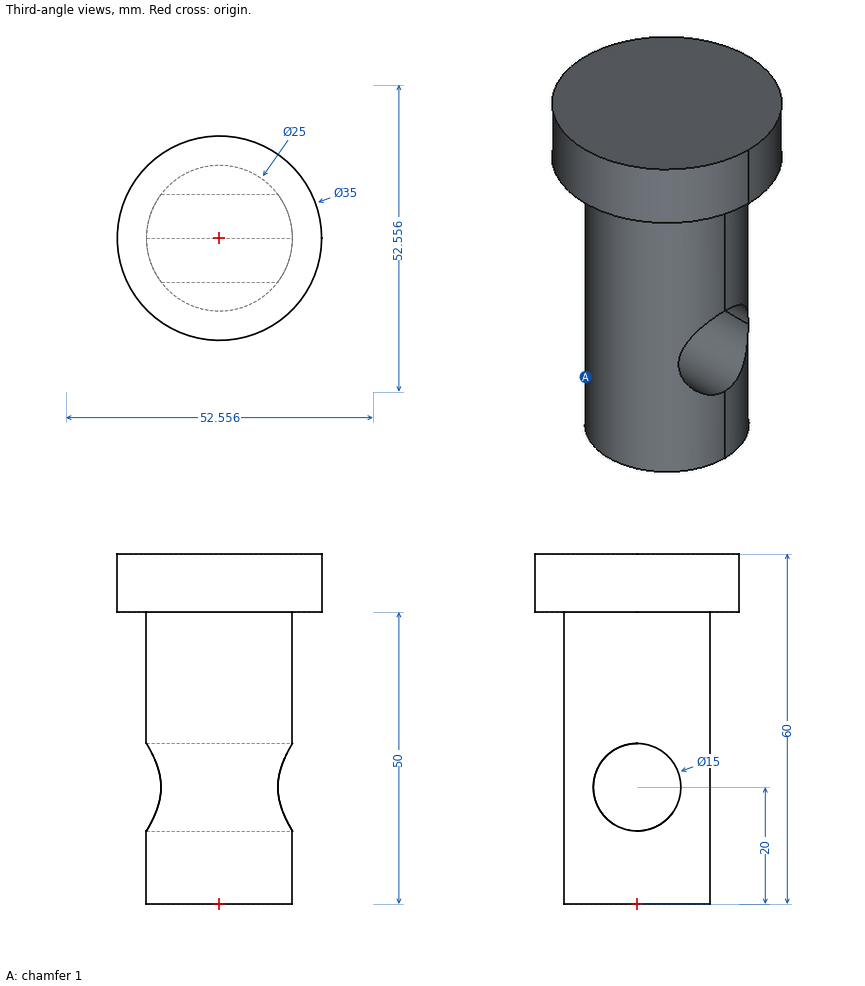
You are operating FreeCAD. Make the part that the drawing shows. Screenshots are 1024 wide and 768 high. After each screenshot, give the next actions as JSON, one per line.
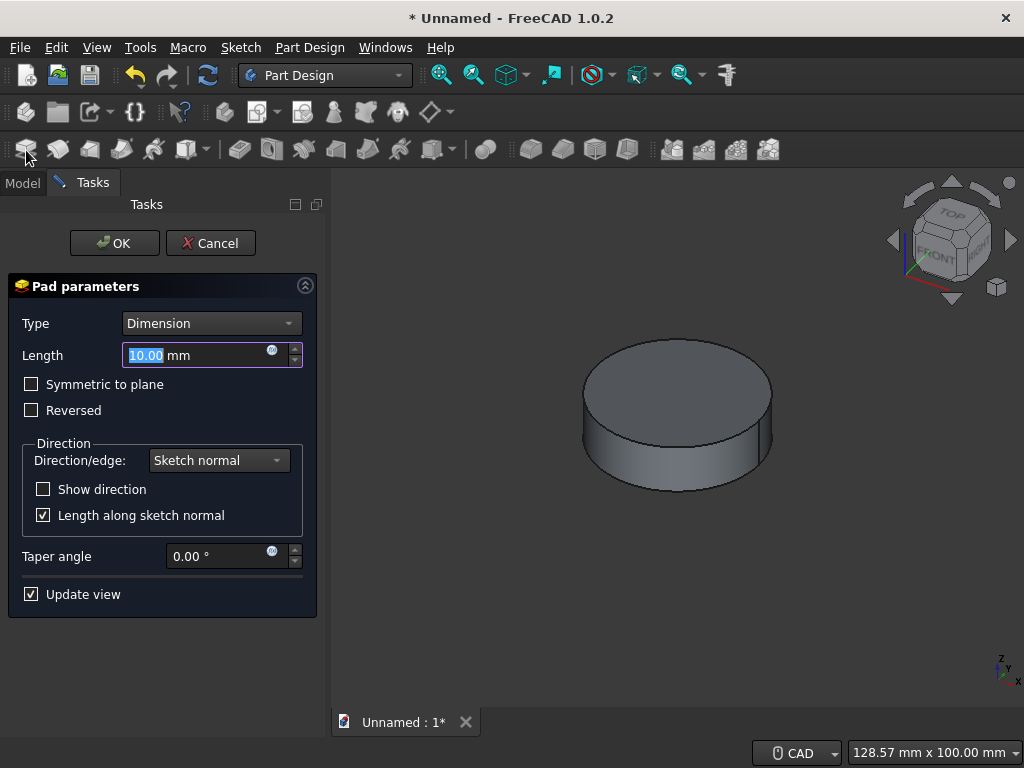
{"action": "type", "text": "60"}
{"action": "key", "text": "Tab"}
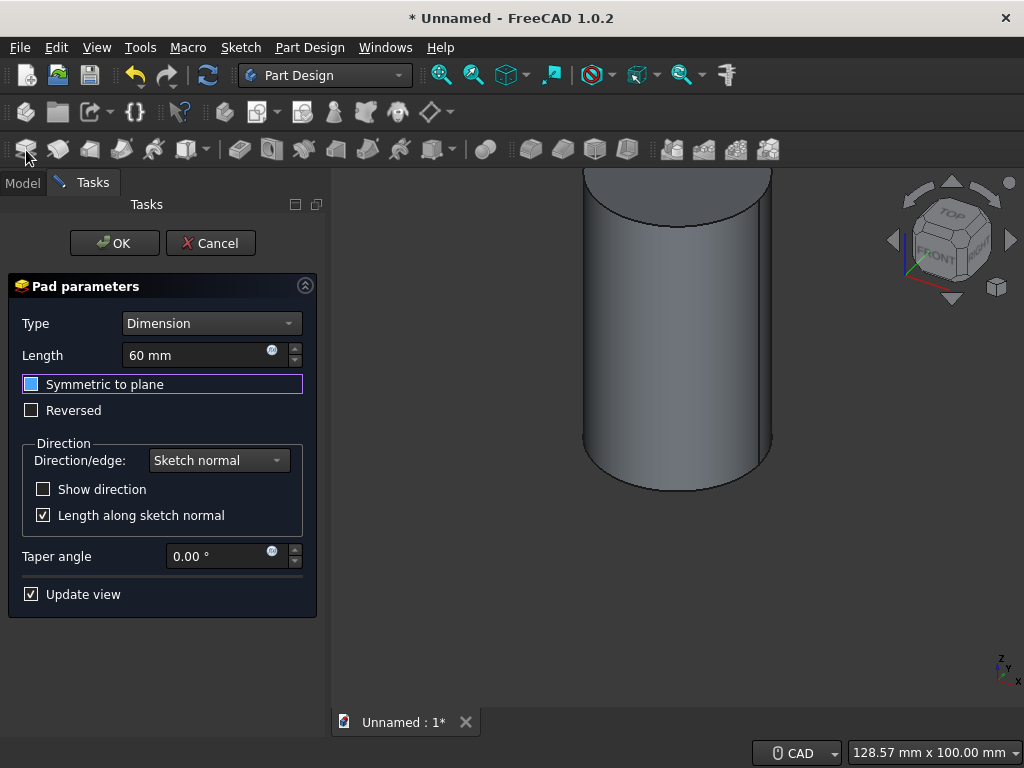
{"action": "left_click", "coordinate": [115, 243]}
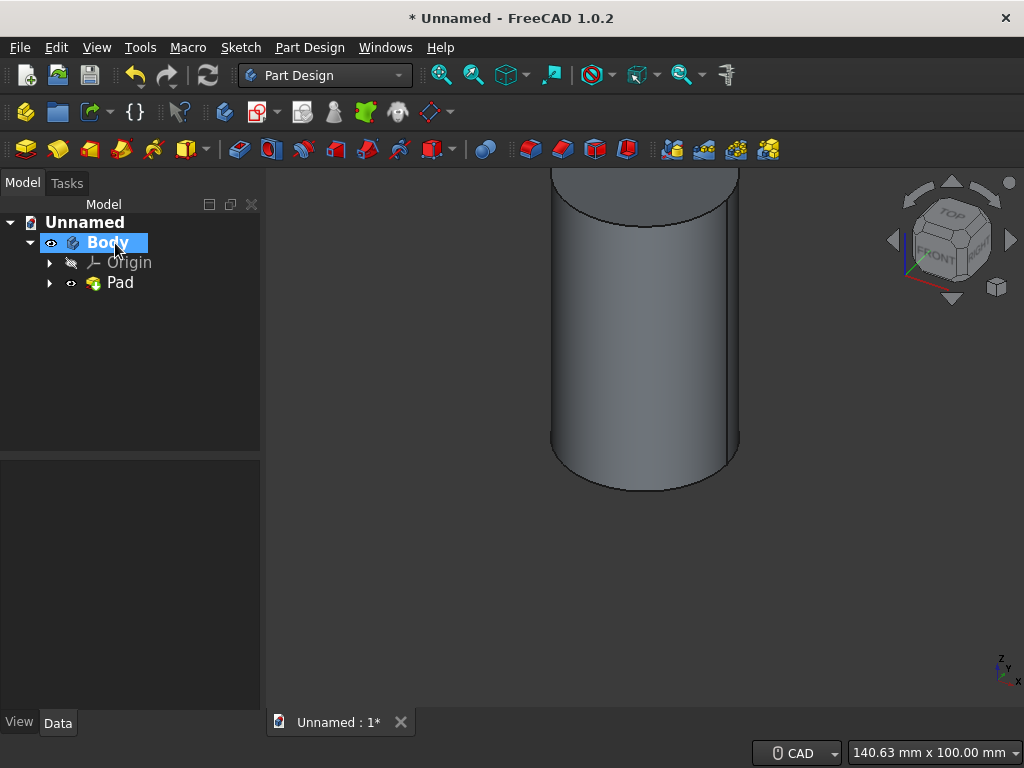
{"action": "left_click", "coordinate": [442, 76]}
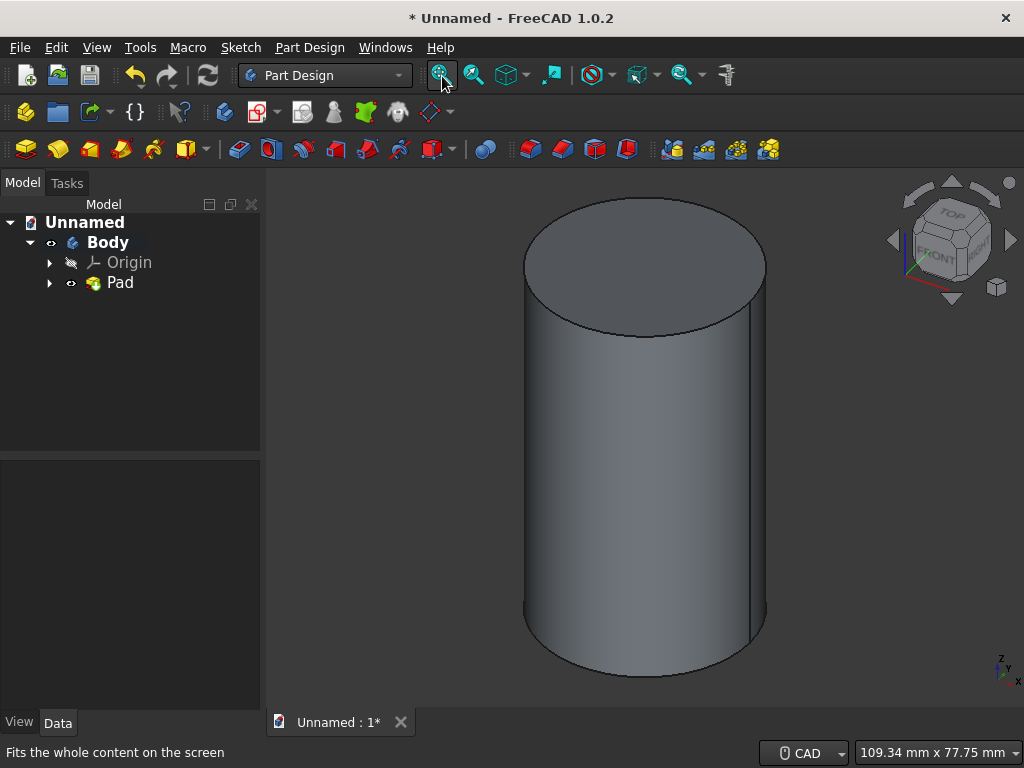
{"action": "key", "text": "0"}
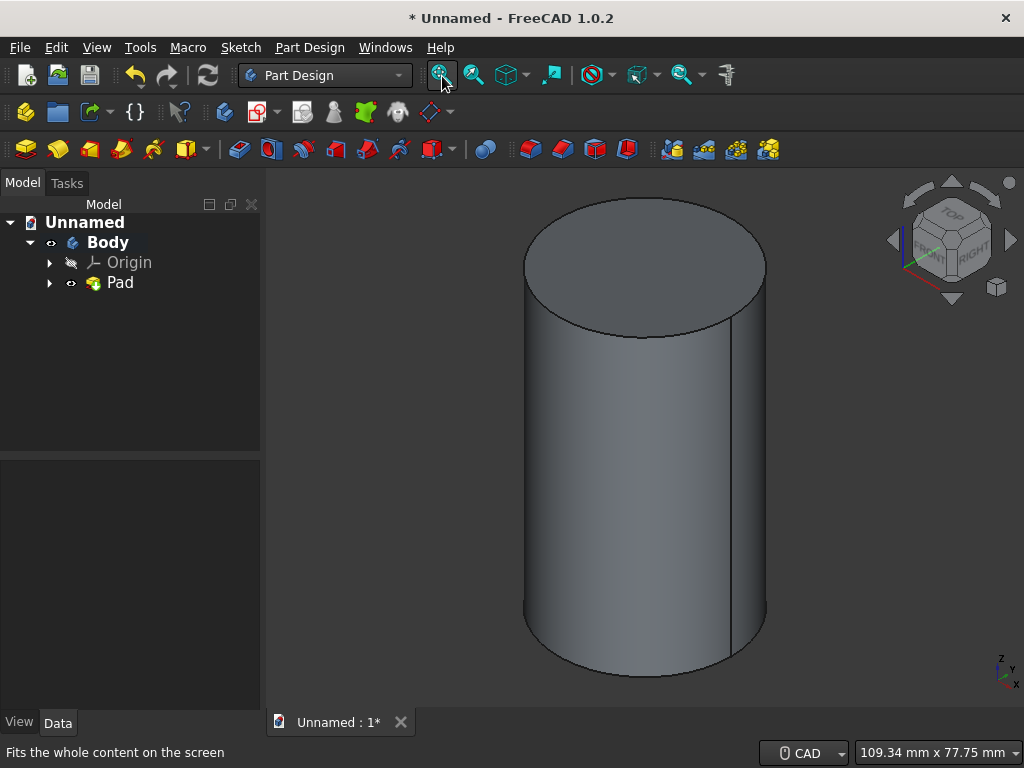
{"action": "left_click", "coordinate": [745, 646]}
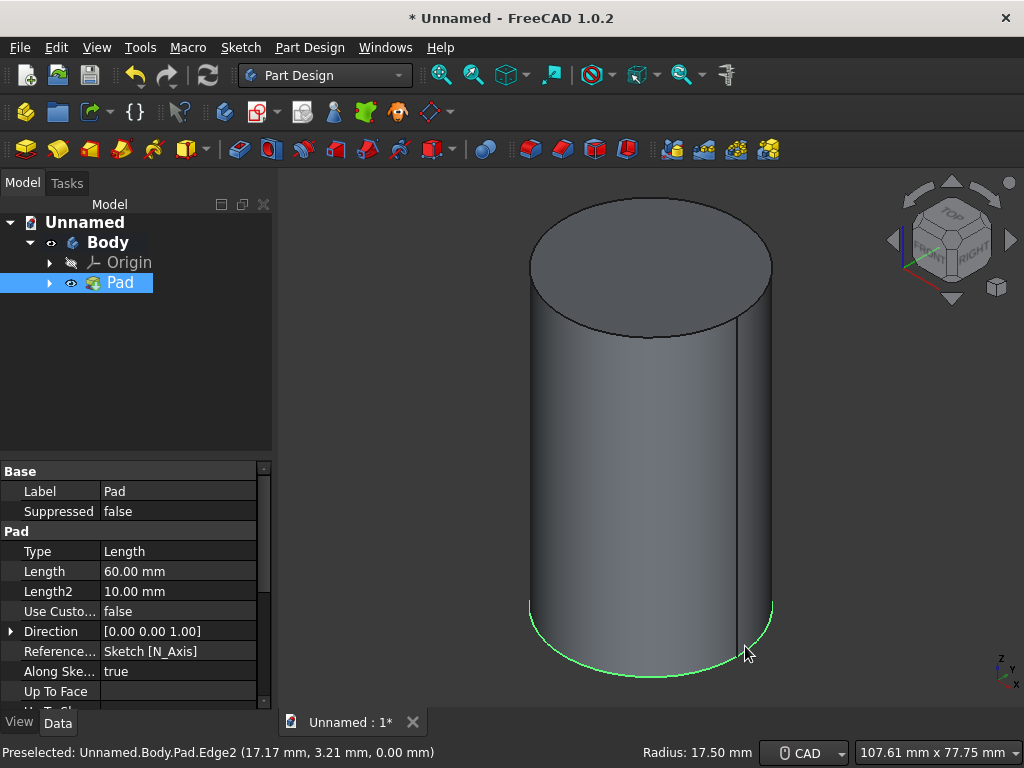
{"action": "left_click", "coordinate": [564, 150]}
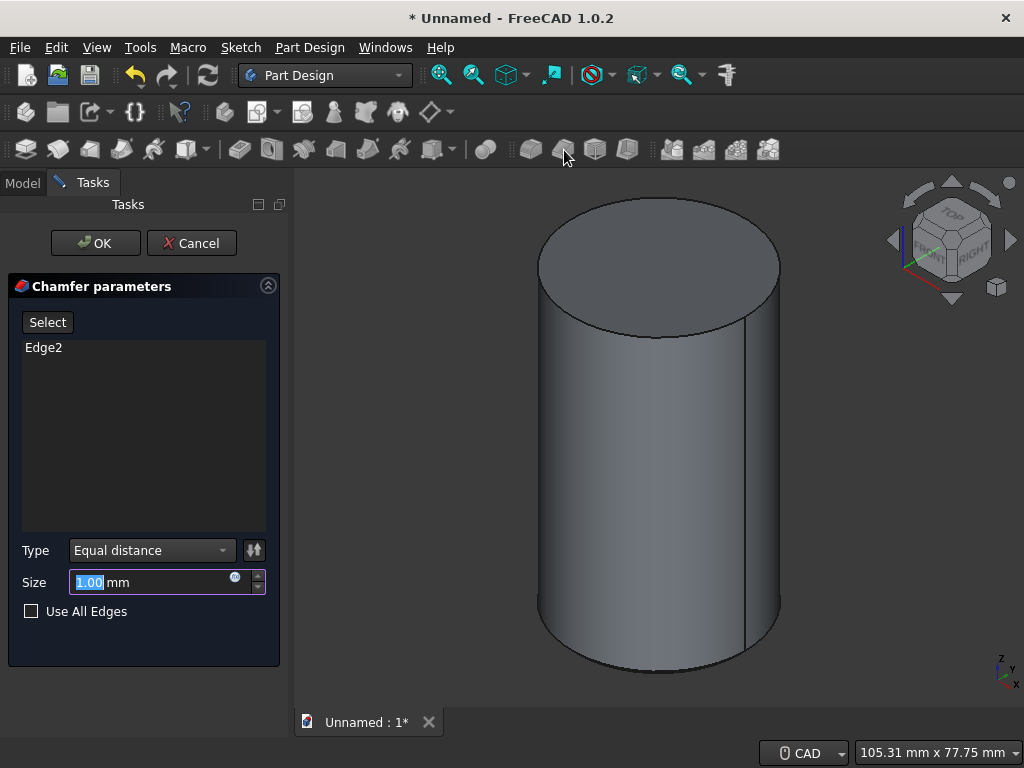
{"action": "type", "text": "1"}
{"action": "key", "text": "Tab"}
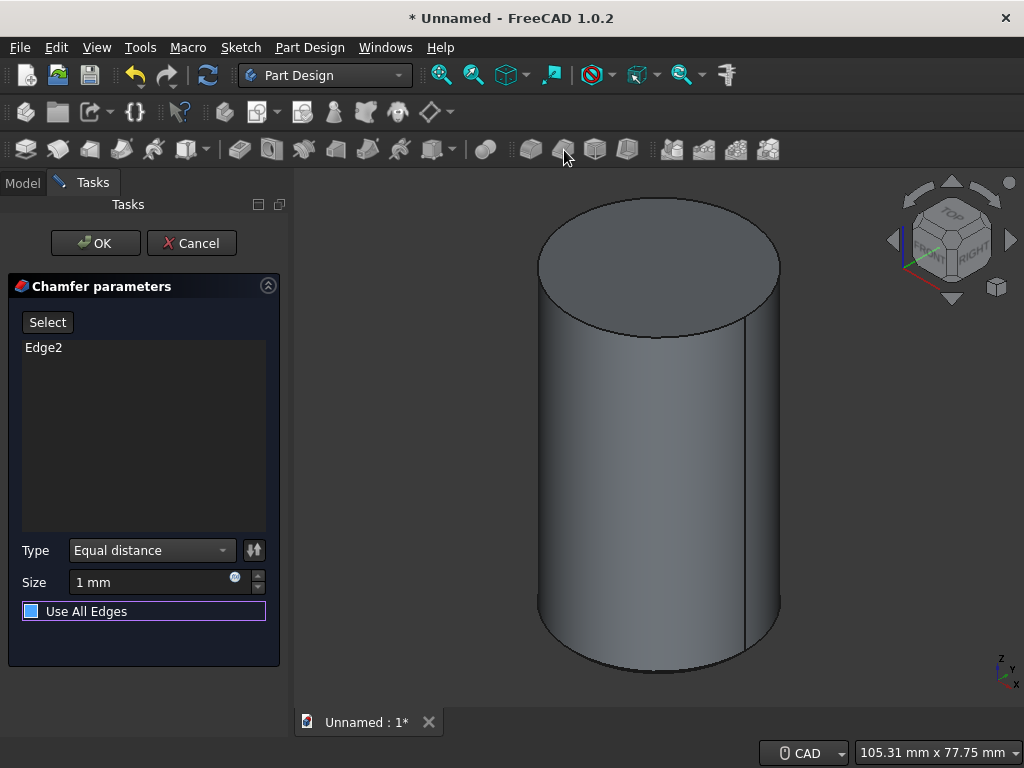
{"action": "left_click", "coordinate": [96, 243]}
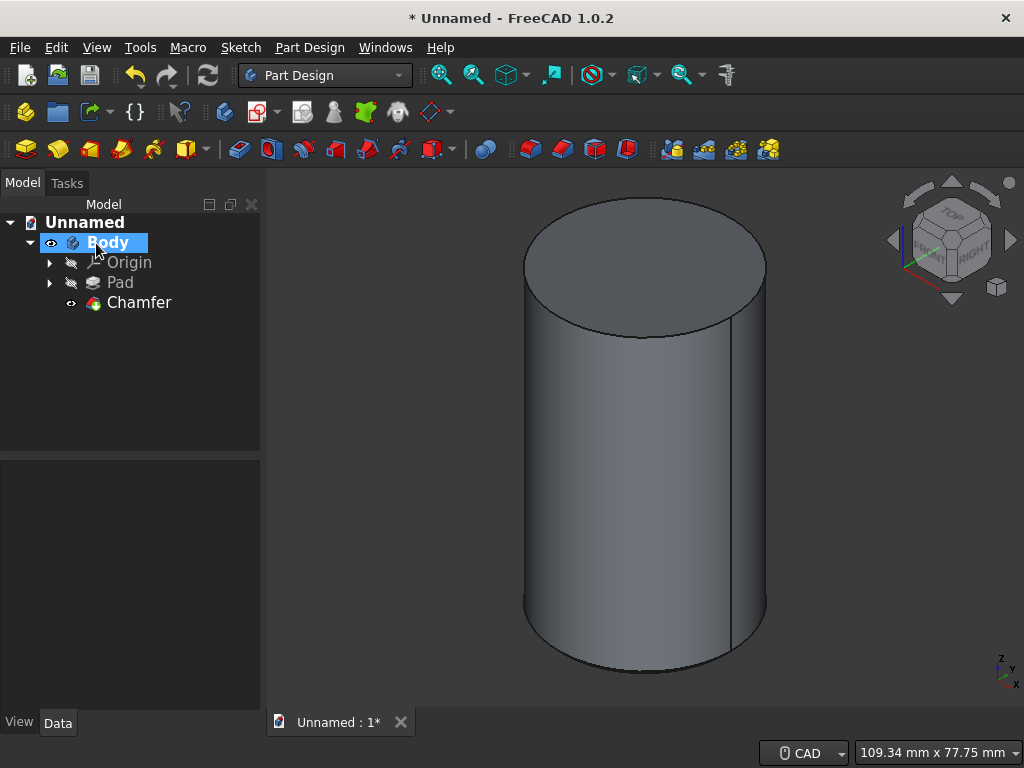
{"action": "left_click", "coordinate": [258, 112]}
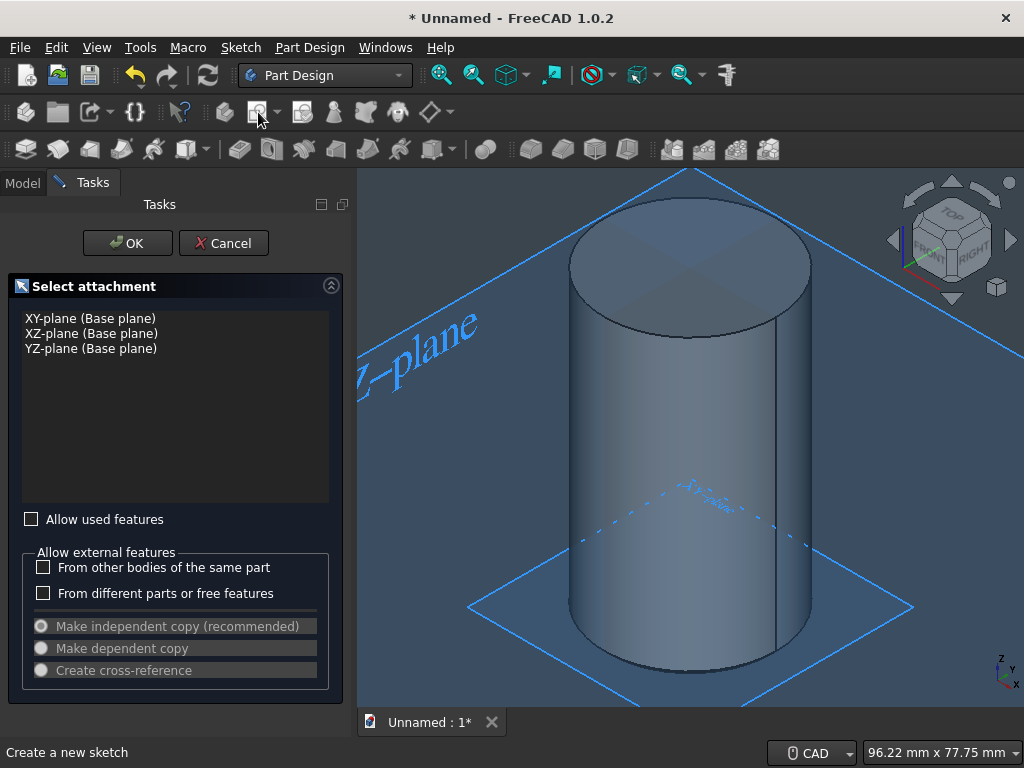
{"action": "left_click", "coordinate": [82, 348]}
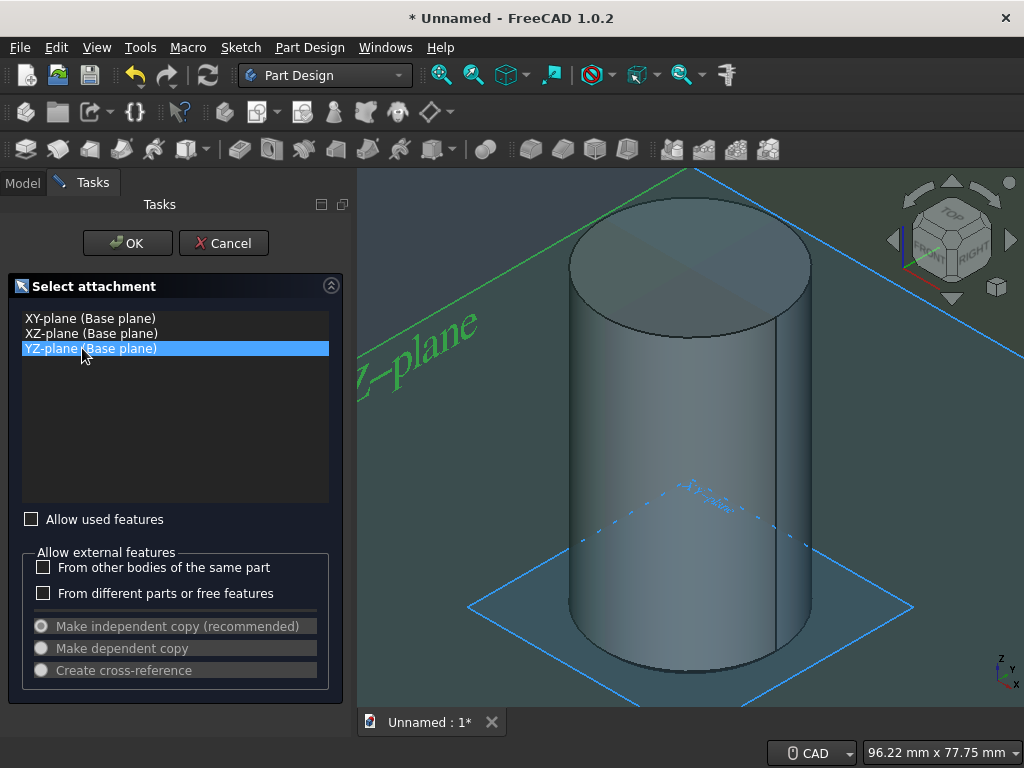
{"action": "left_click", "coordinate": [128, 243]}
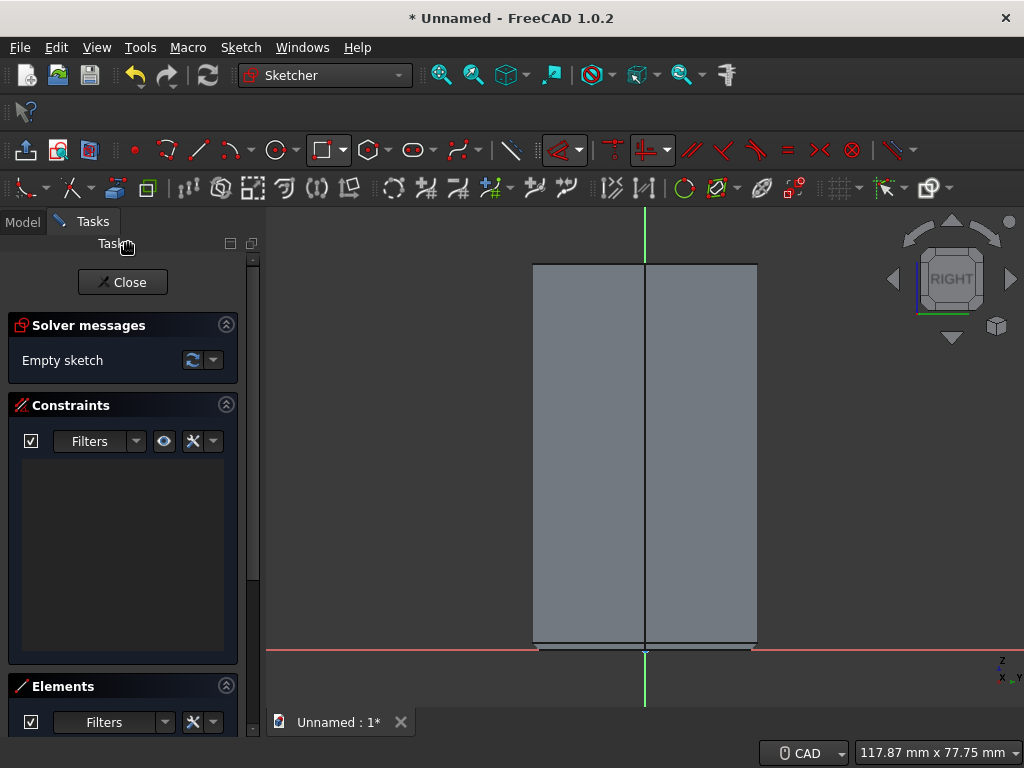
{"action": "key", "text": "q s"}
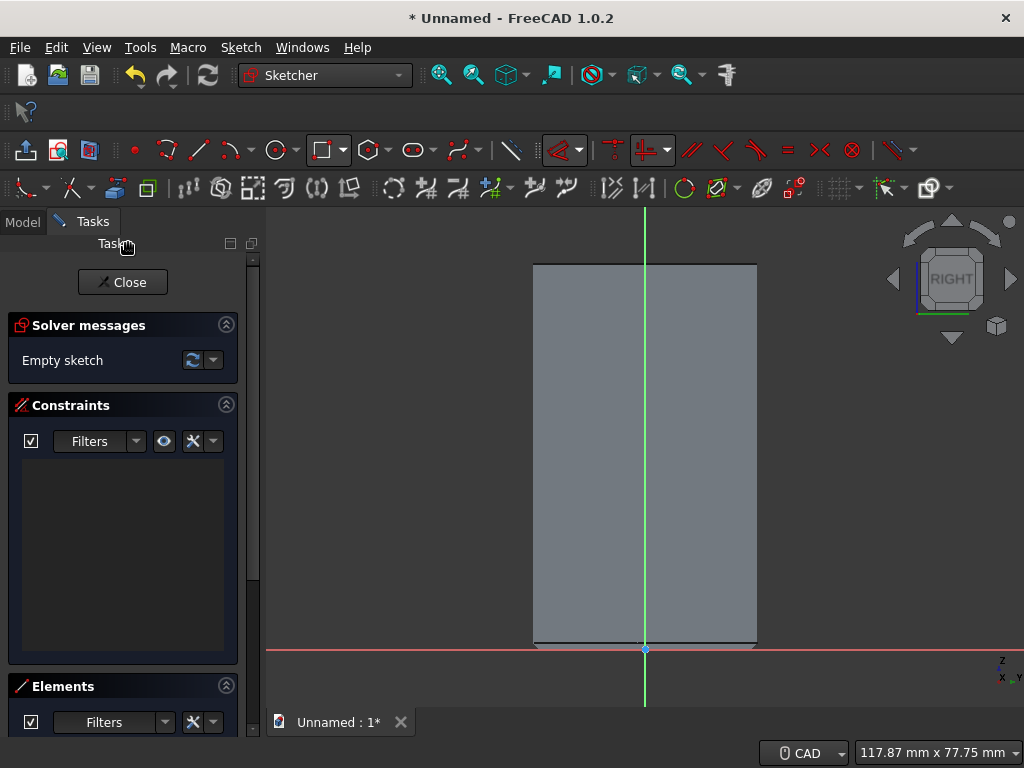
{"action": "scroll", "coordinate": [728, 679], "scroll_direction": "up", "scroll_amount": 3}